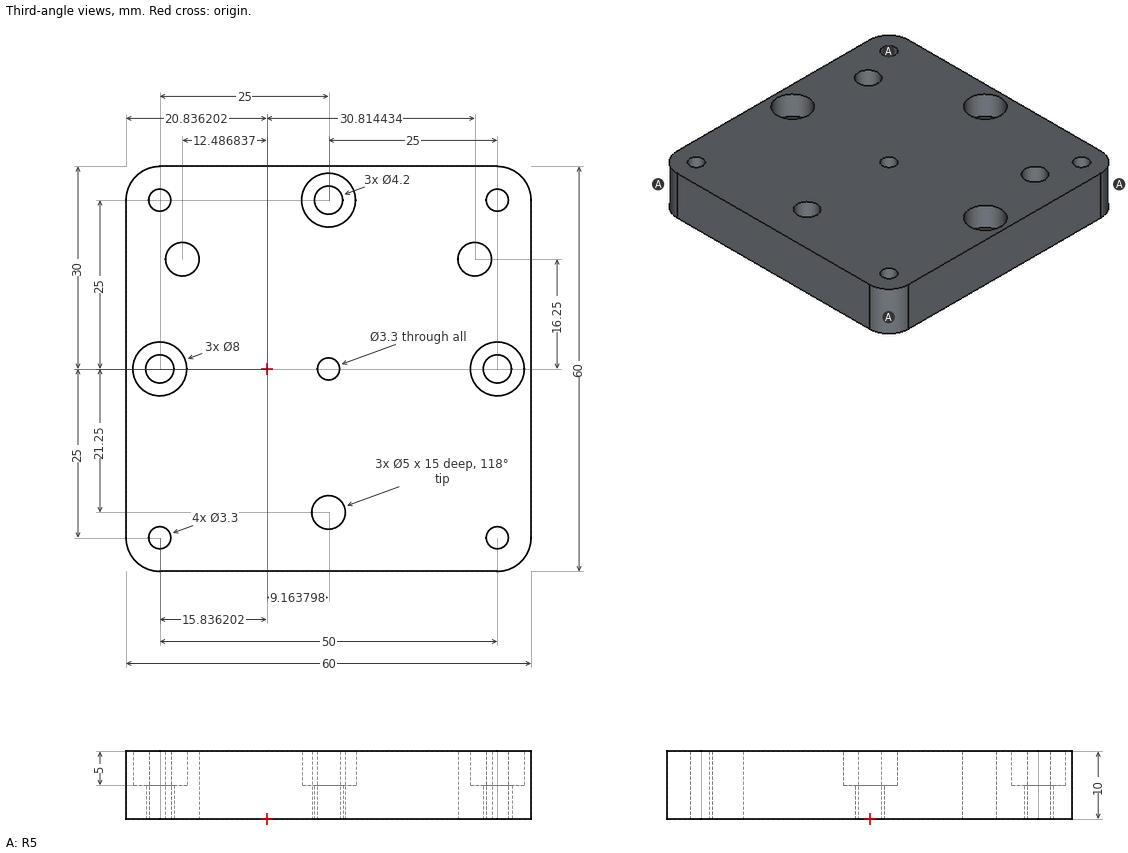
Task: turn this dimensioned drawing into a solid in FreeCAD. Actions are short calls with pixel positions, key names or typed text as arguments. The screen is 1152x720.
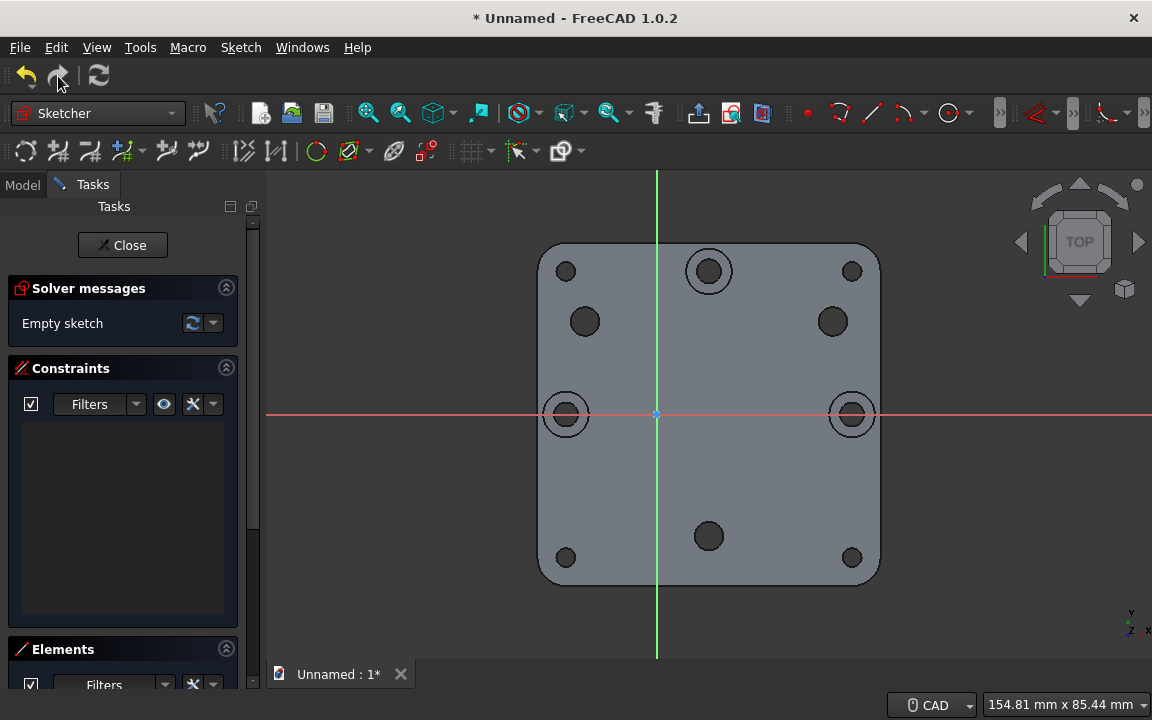
scroll(713, 414, up, 14)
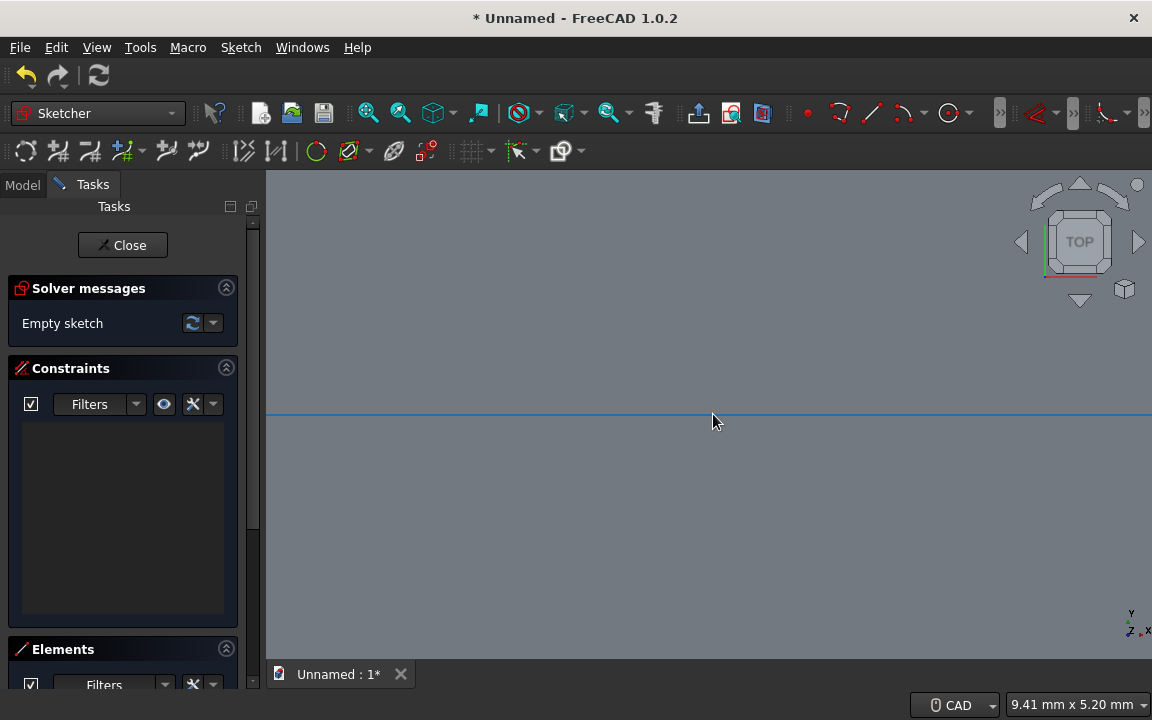
click(950, 114)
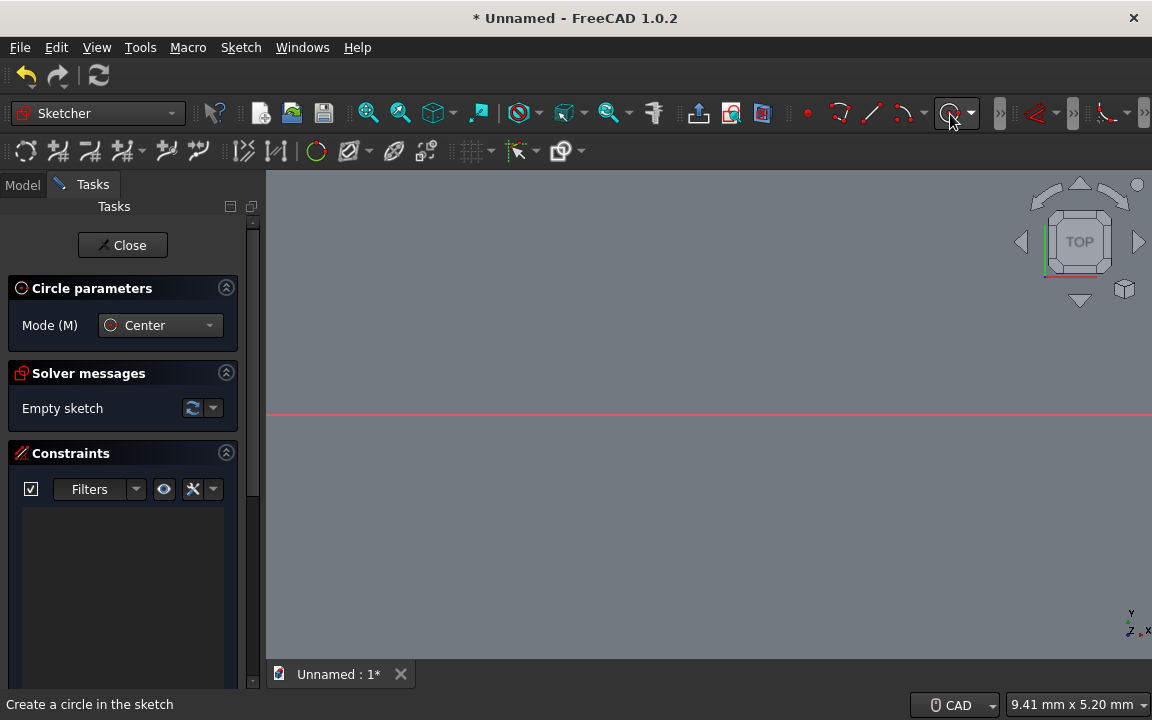
click(639, 414)
move(749, 305)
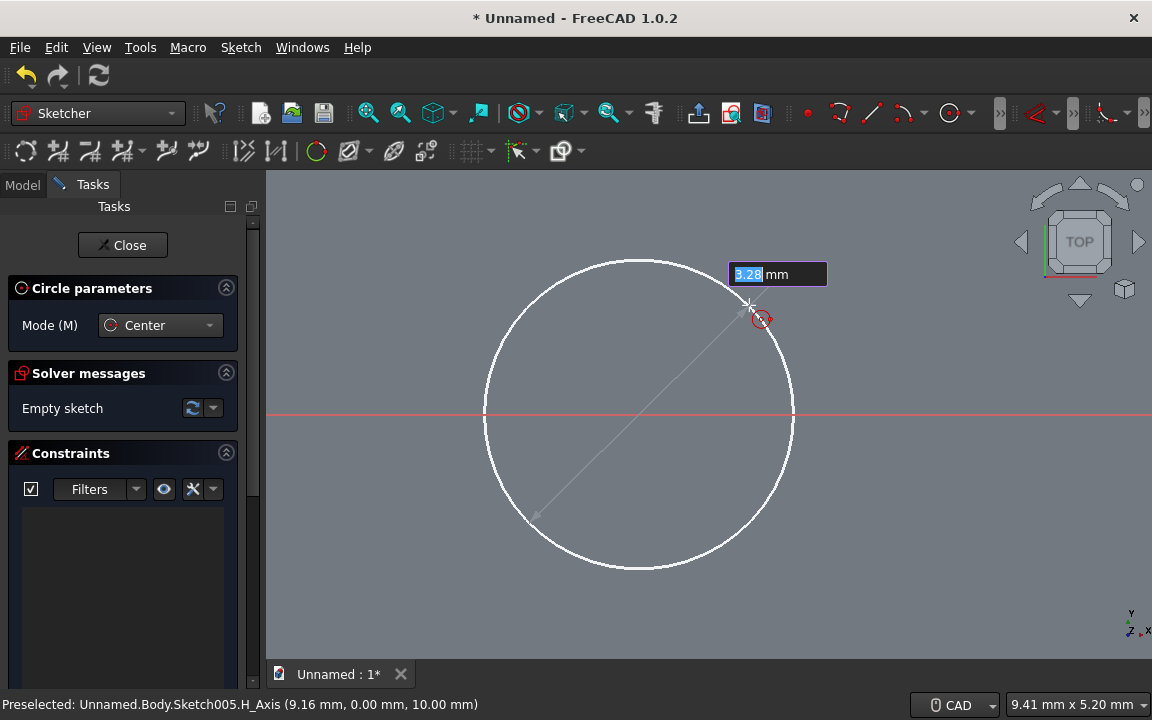
text(3.3)
key(Return)
key(Escape)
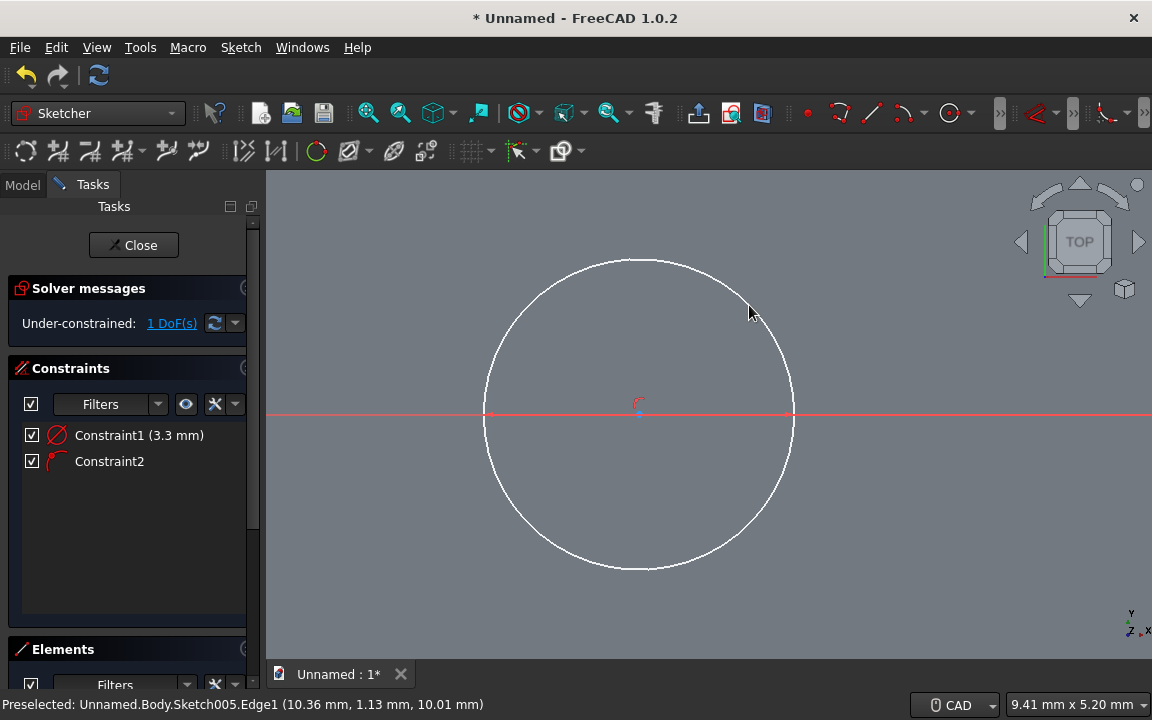
click(1036, 114)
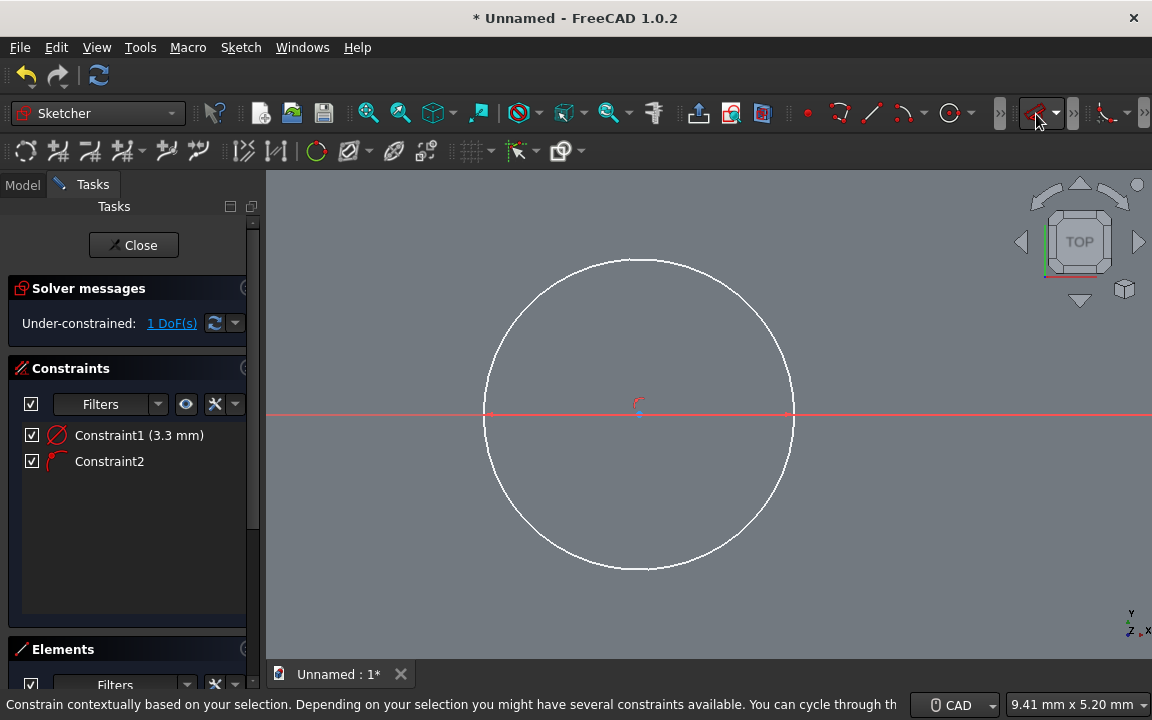
click(639, 414)
click(466, 448)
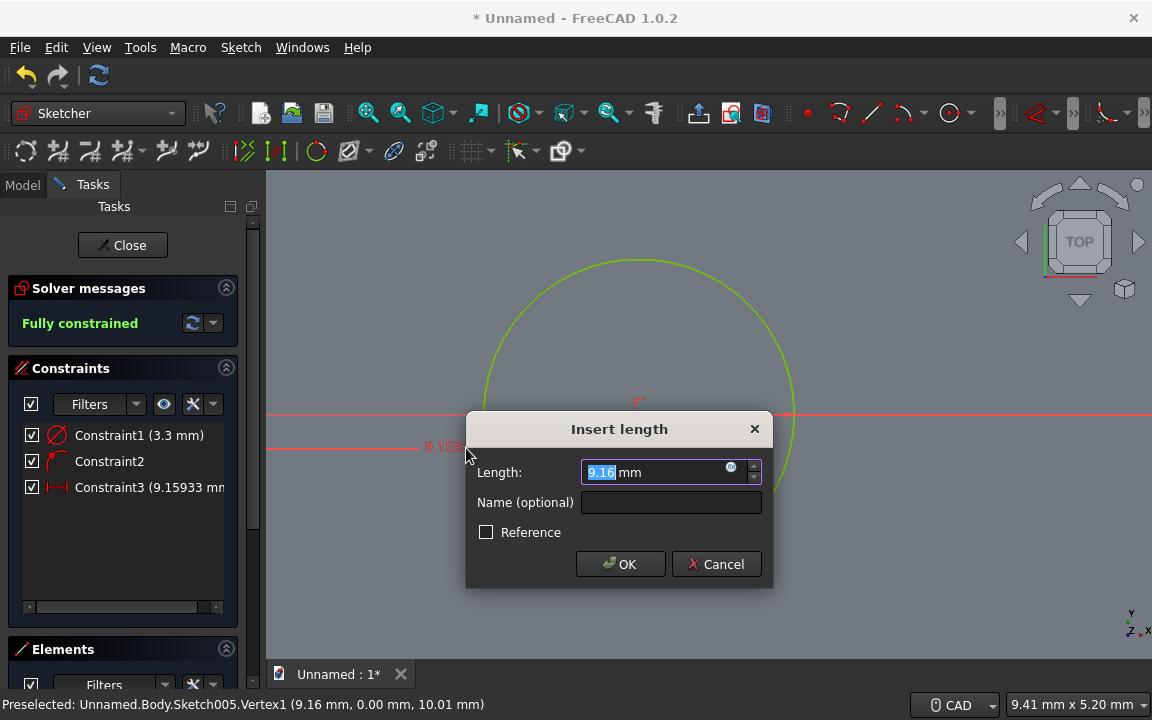
text(9.163798)
key(Return)
key(Escape)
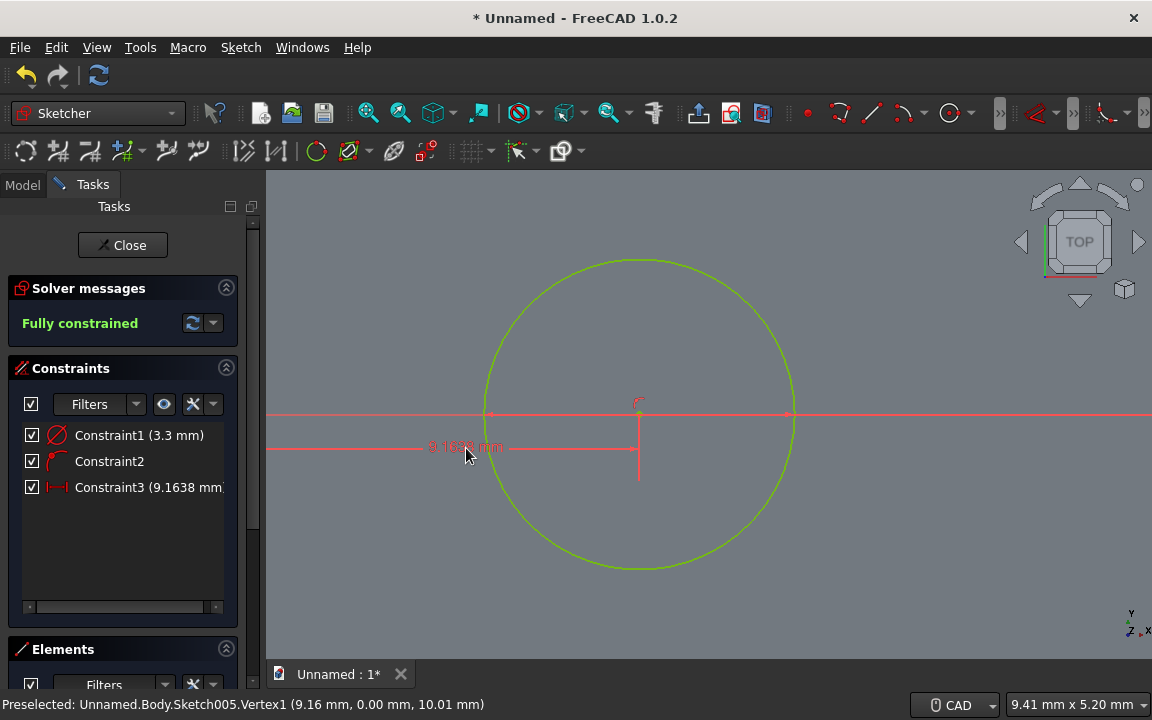
click(123, 245)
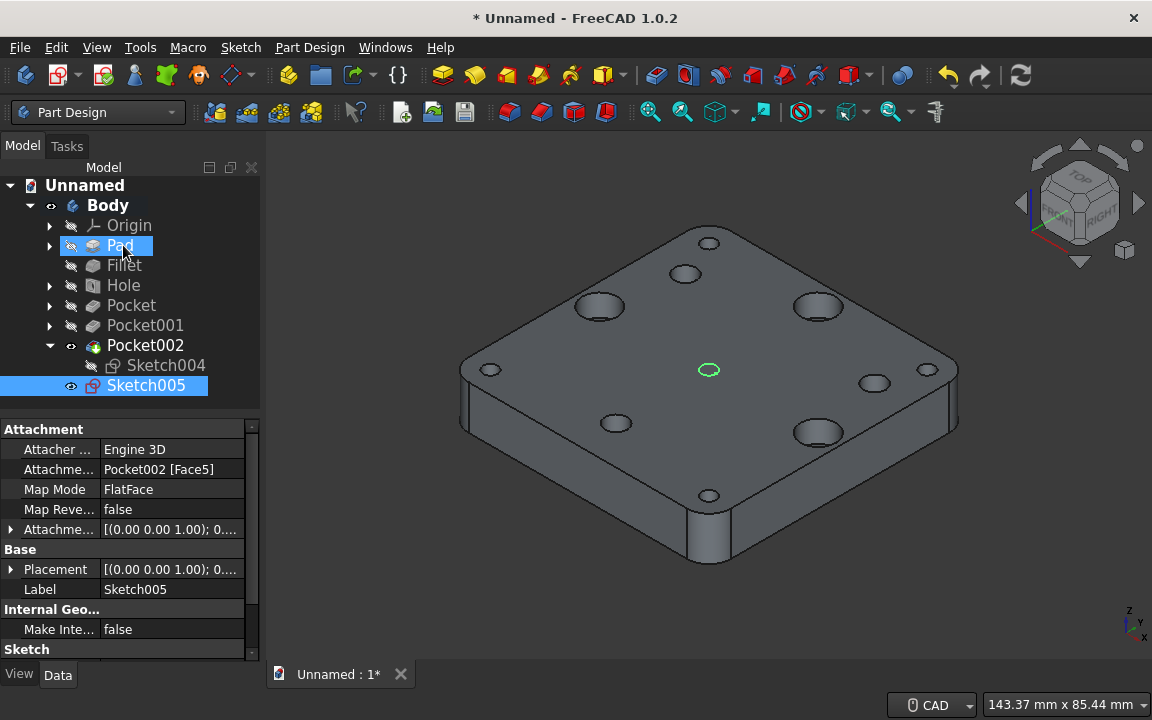
click(690, 76)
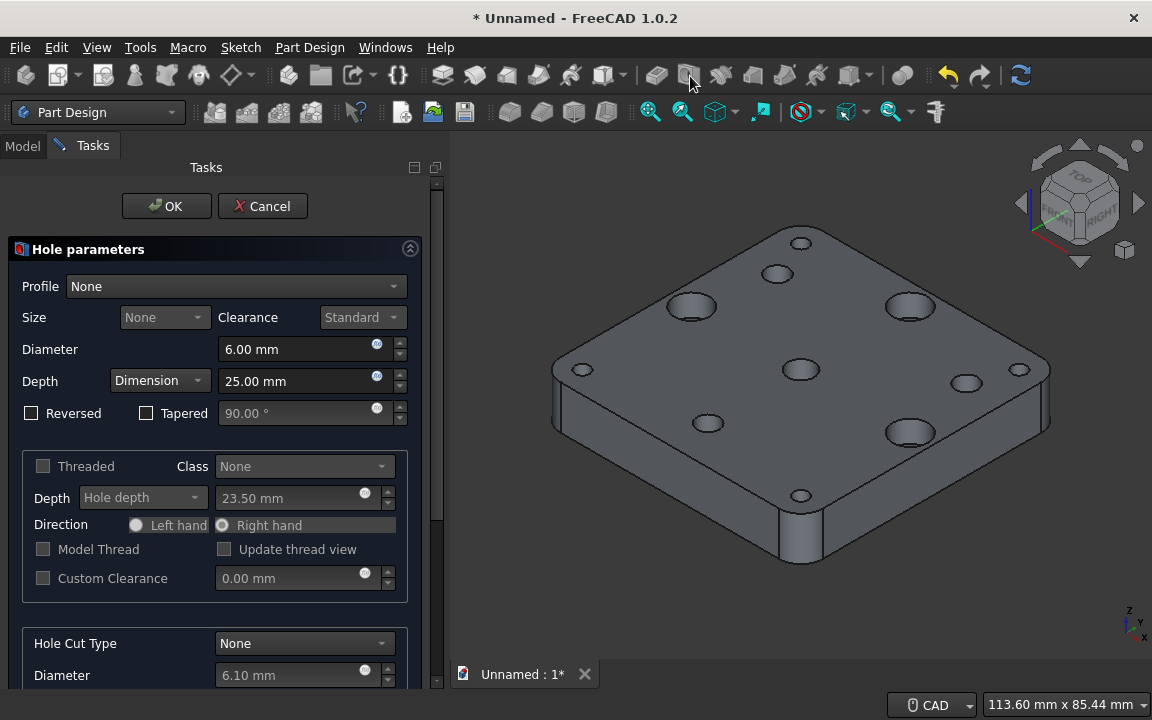
triple_click(305, 349)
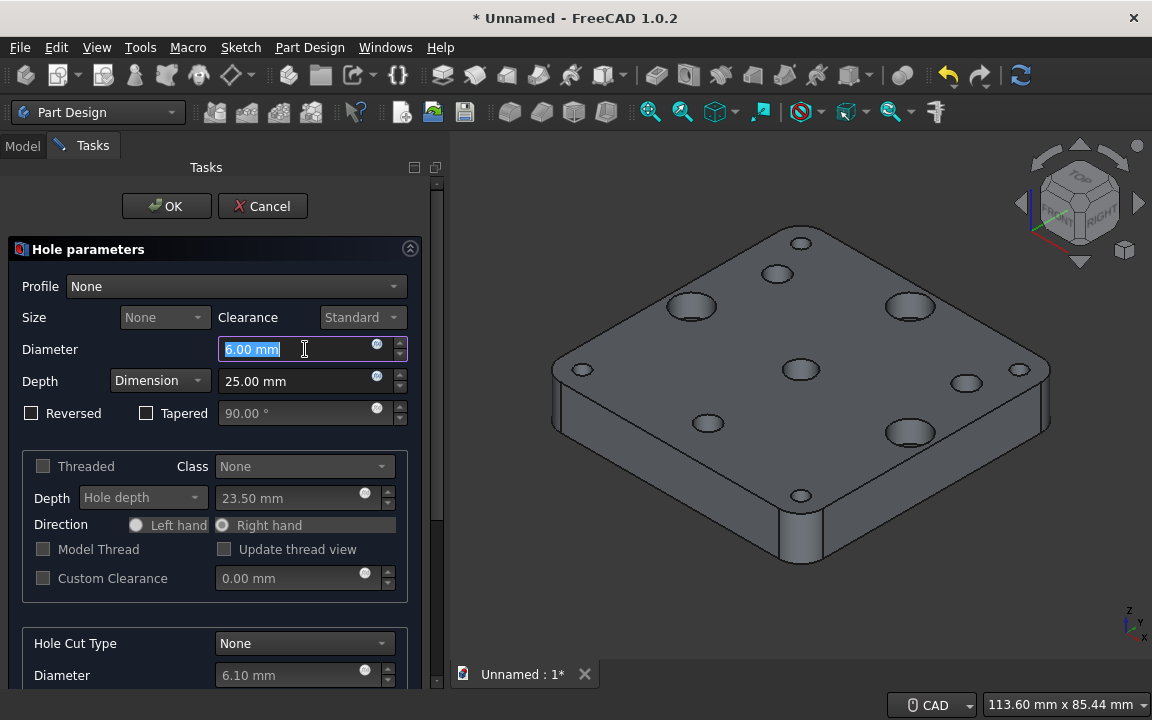
text(3.3)
key(Tab)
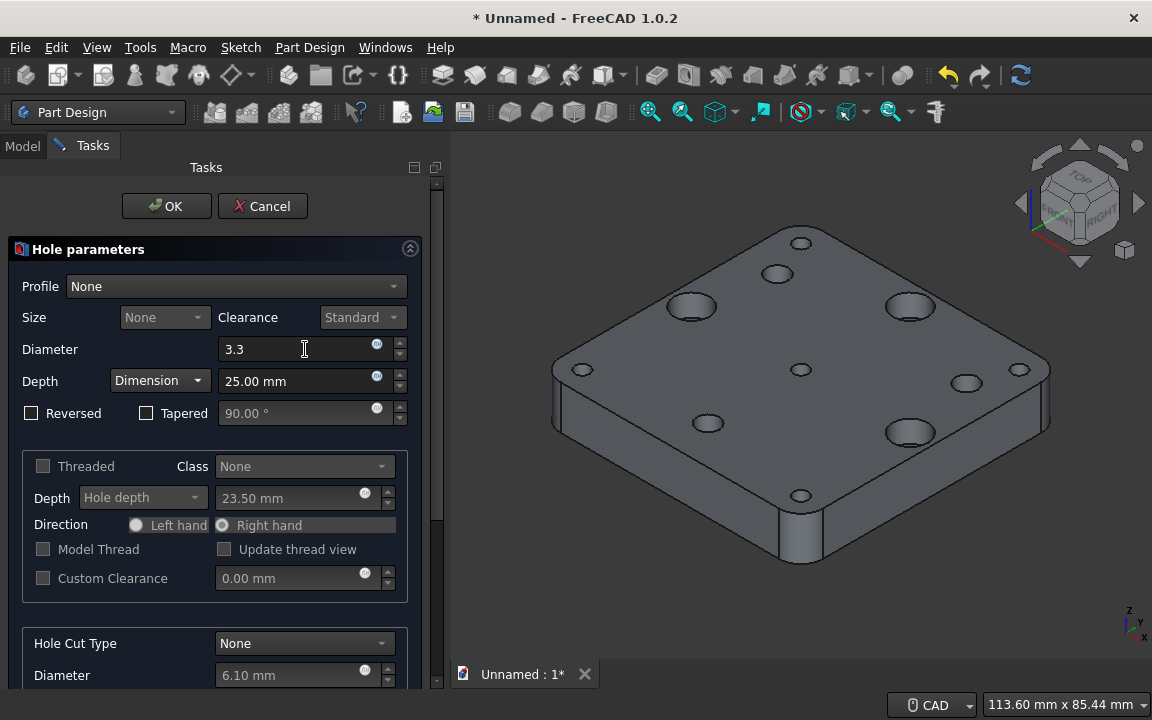
click(161, 380)